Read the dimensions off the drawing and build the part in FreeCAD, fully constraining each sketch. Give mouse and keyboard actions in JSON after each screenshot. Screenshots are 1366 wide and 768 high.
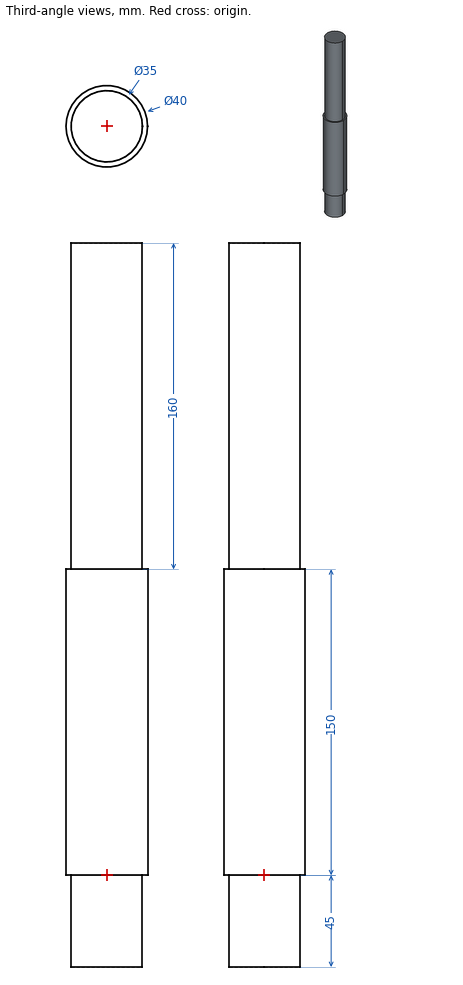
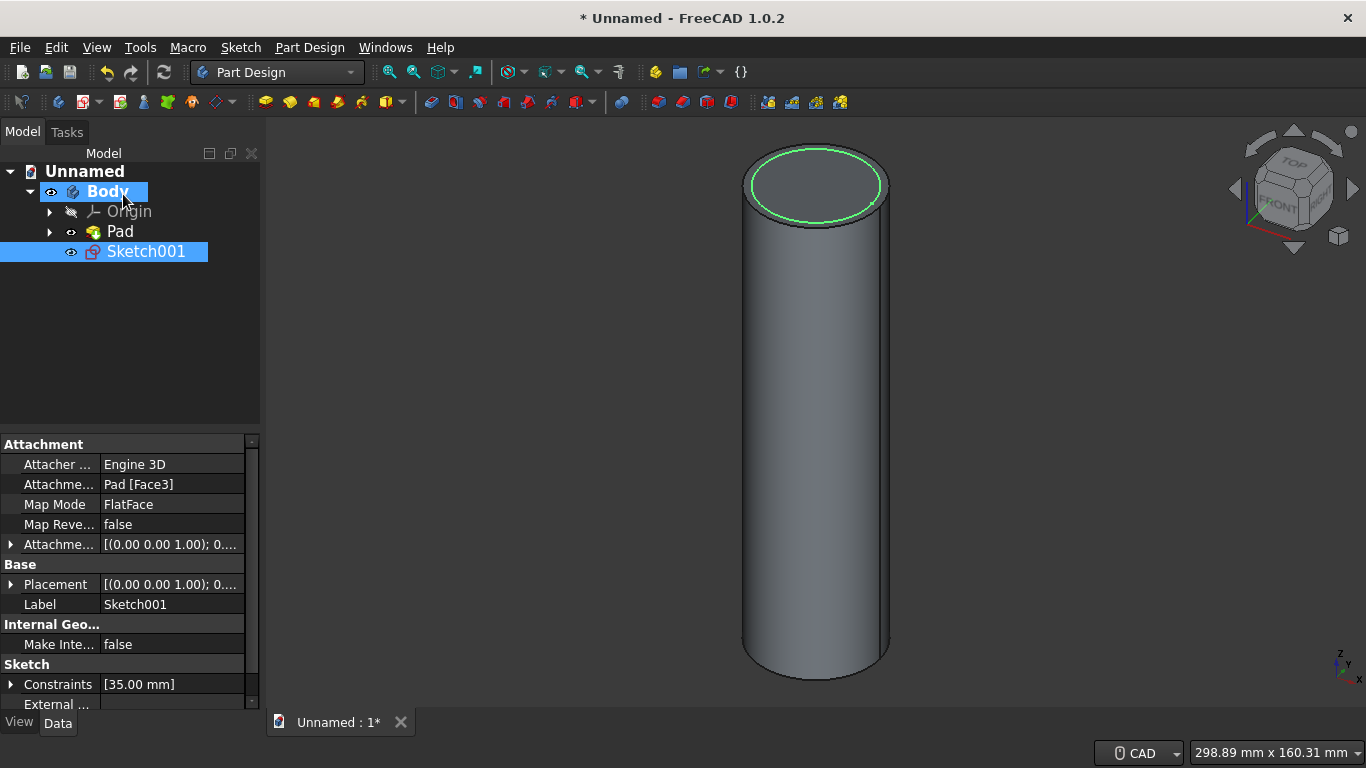
{"action": "left_click", "coordinate": [266, 102]}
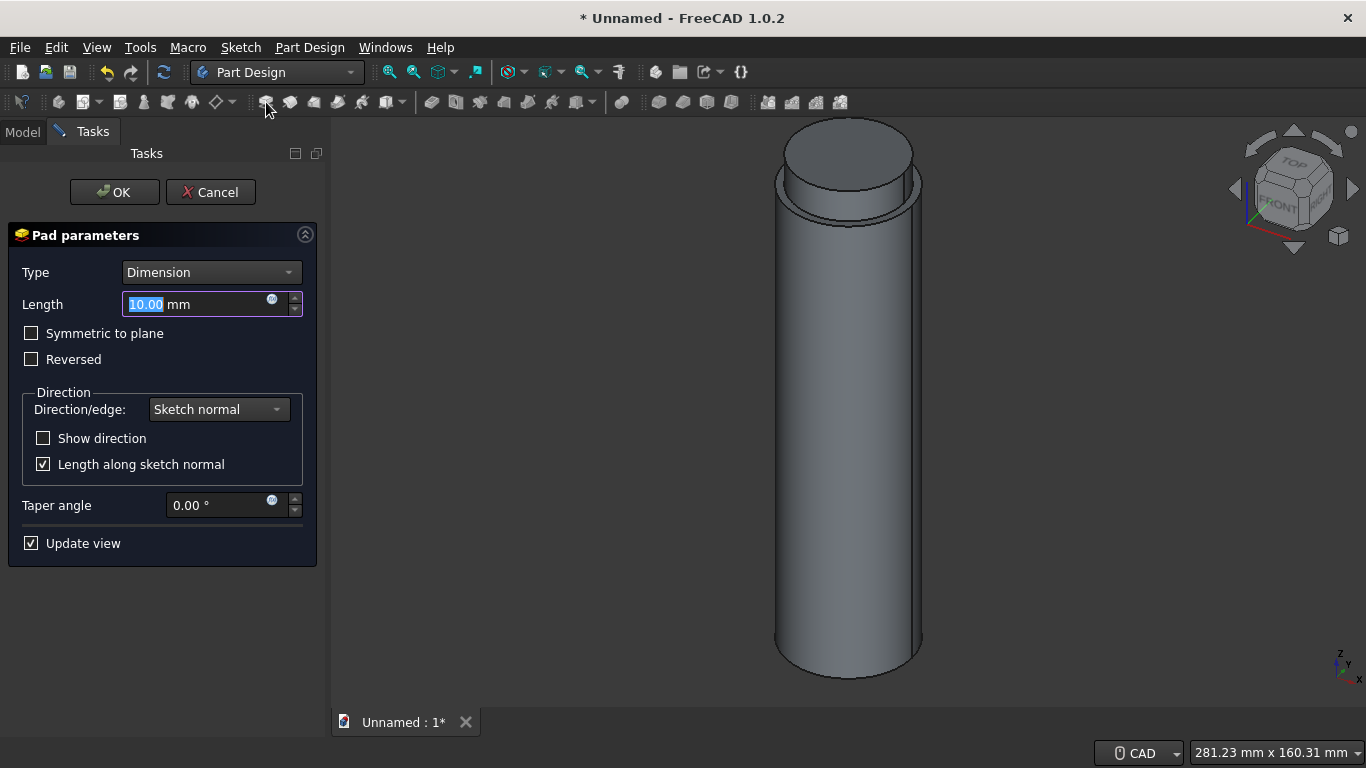
{"action": "type", "text": "160"}
{"action": "key", "text": "Tab"}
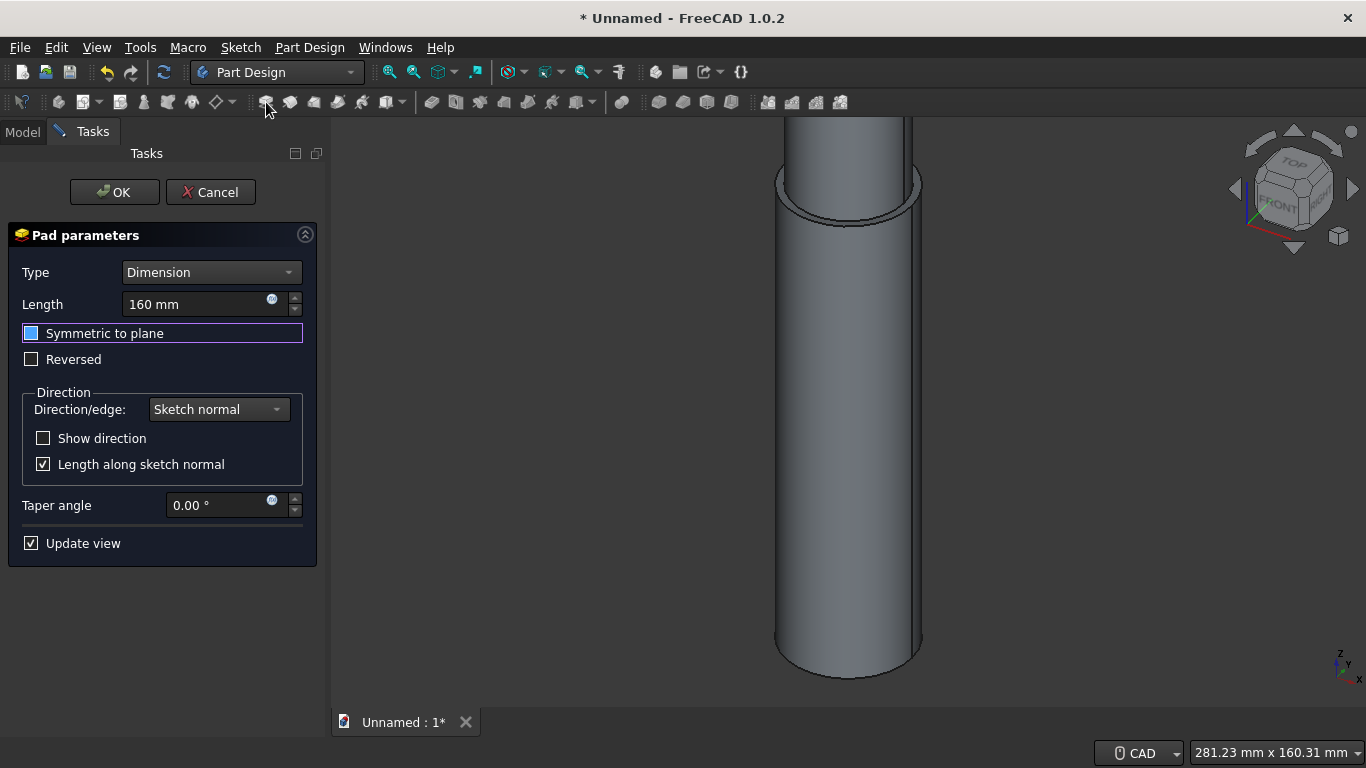
{"action": "left_click", "coordinate": [115, 192]}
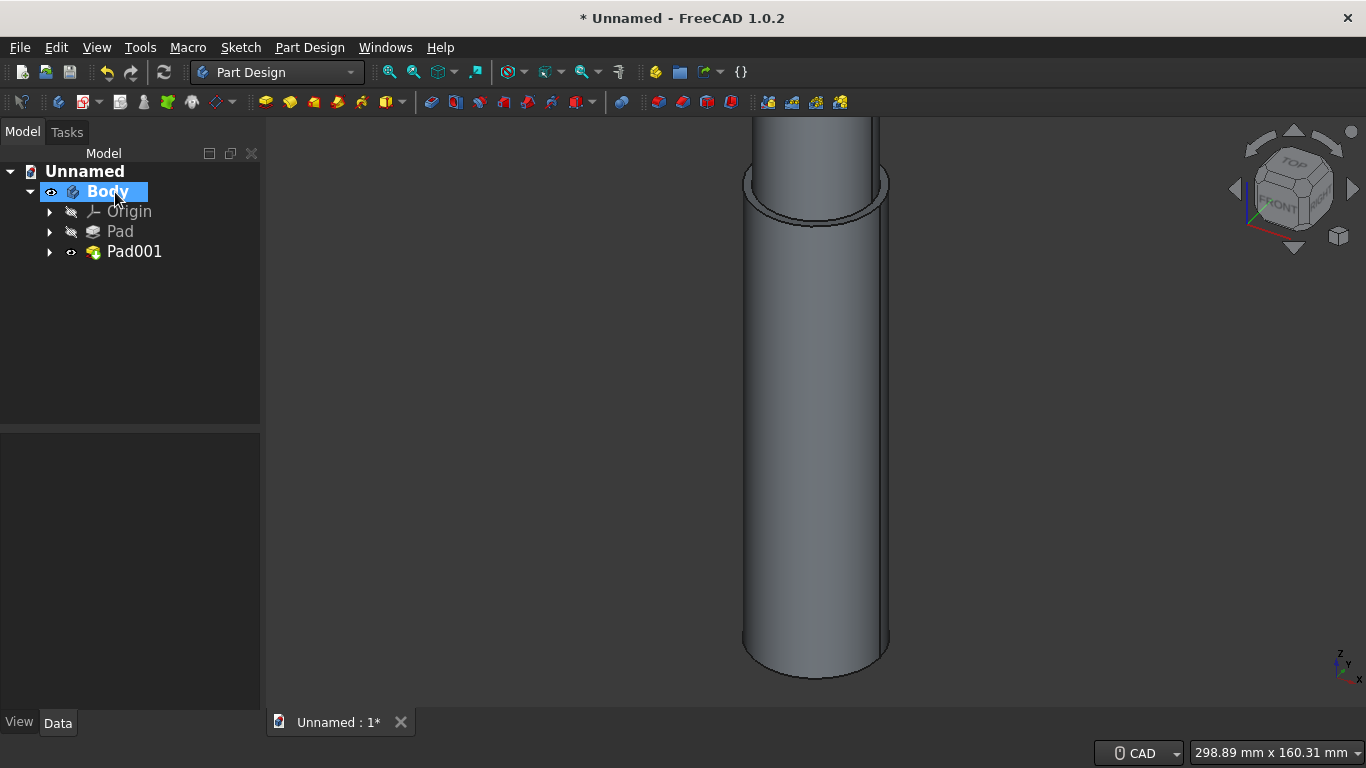
{"action": "left_click", "coordinate": [390, 72]}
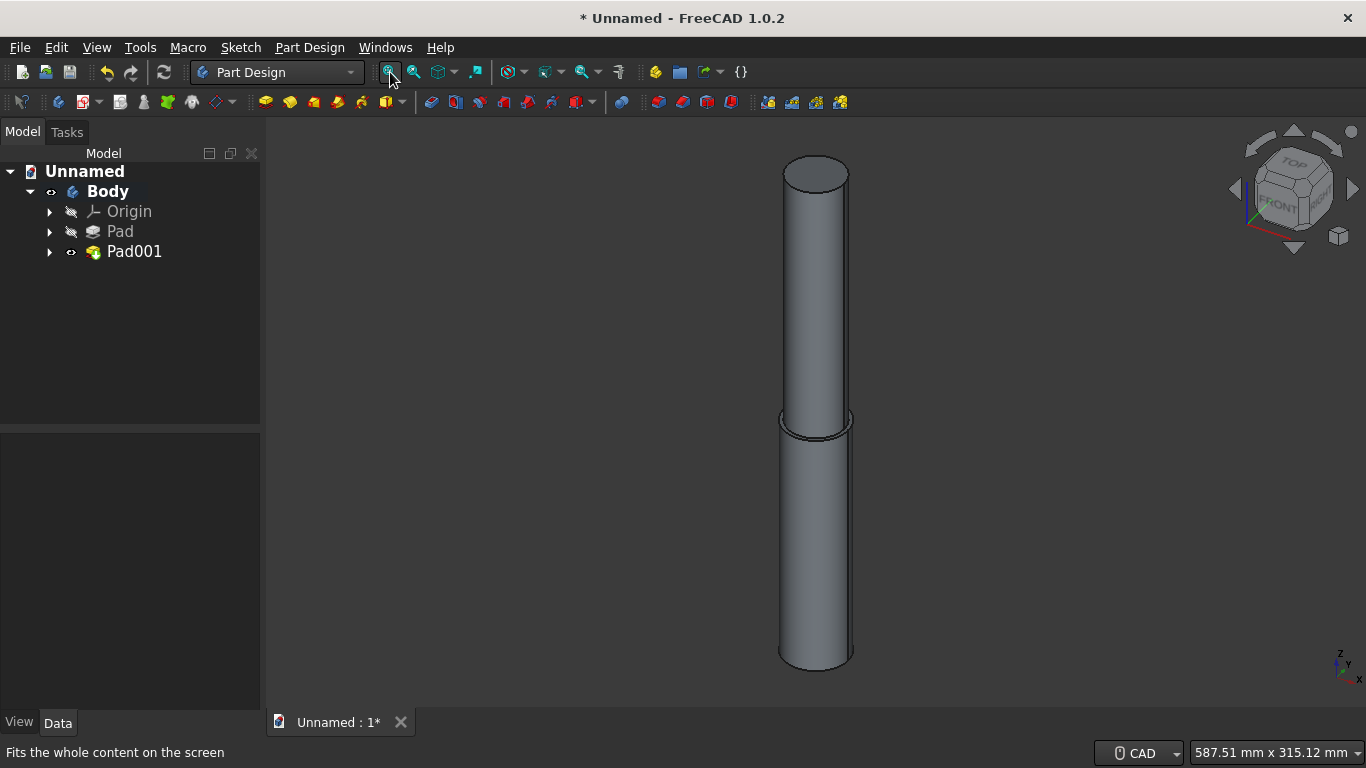
{"action": "left_click", "coordinate": [50, 212]}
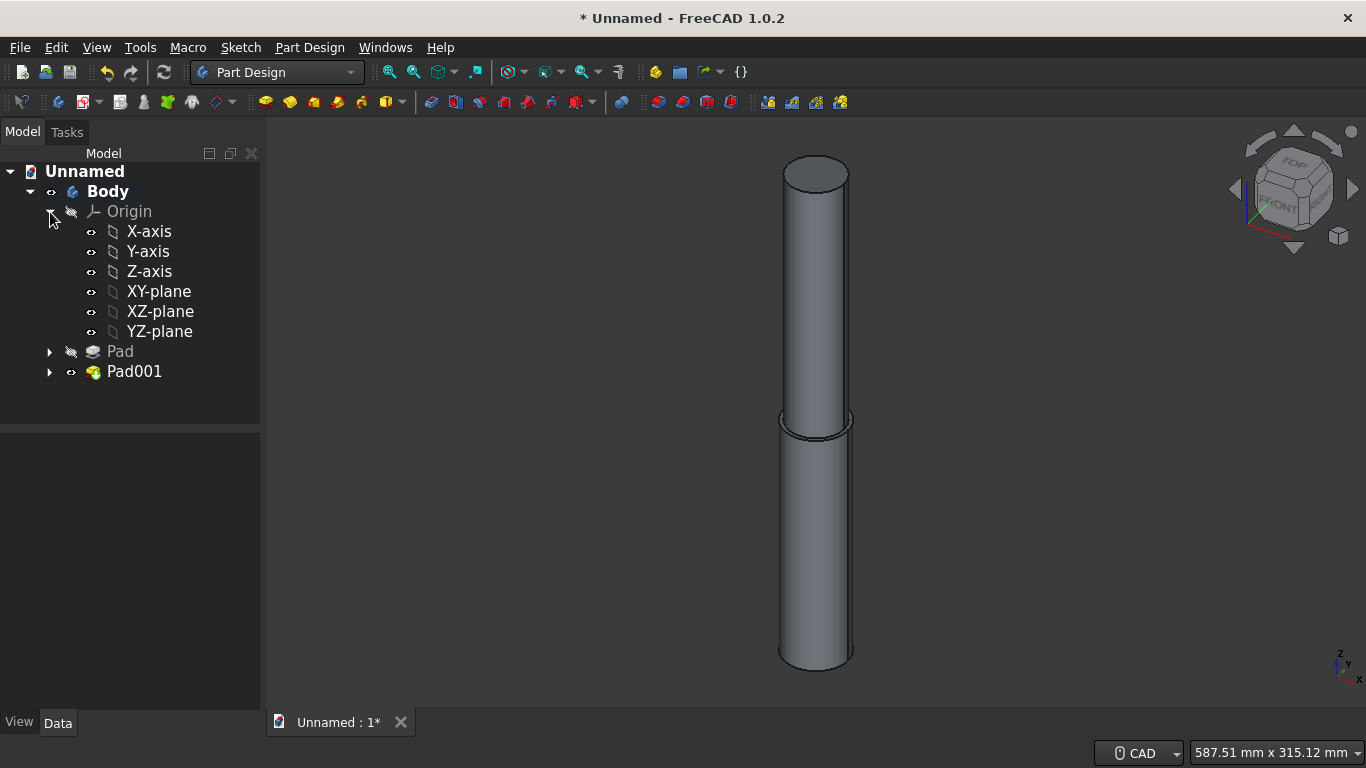
{"action": "left_click", "coordinate": [136, 292]}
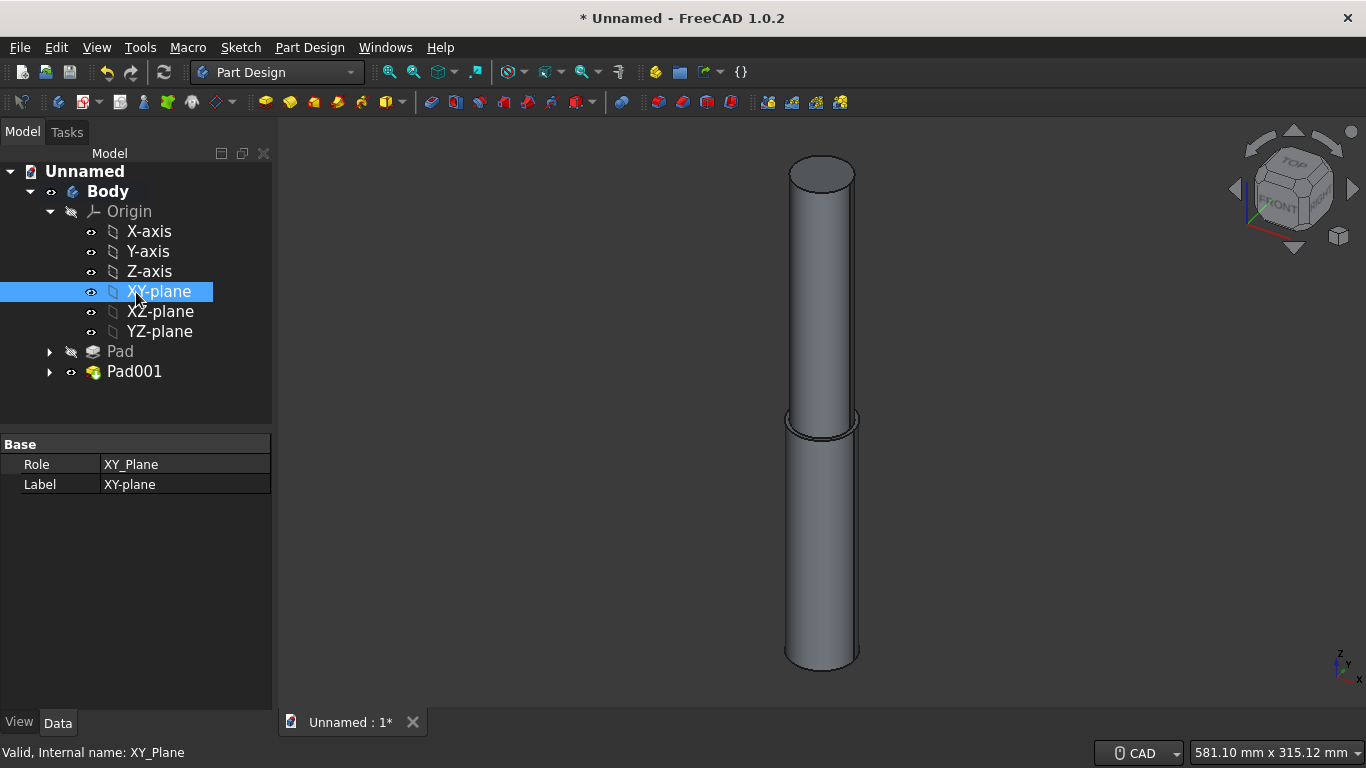
{"action": "left_click", "coordinate": [216, 102]}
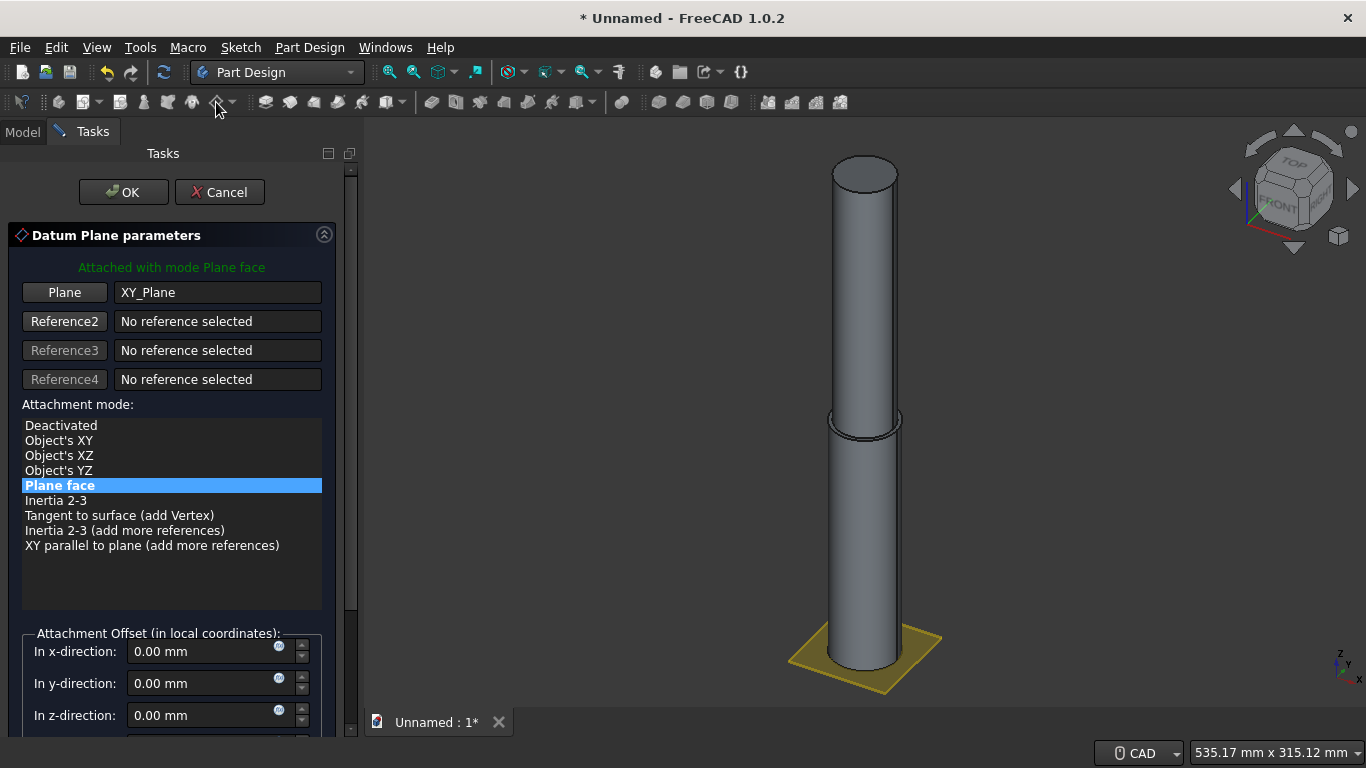
{"action": "triple_click", "coordinate": [210, 715]}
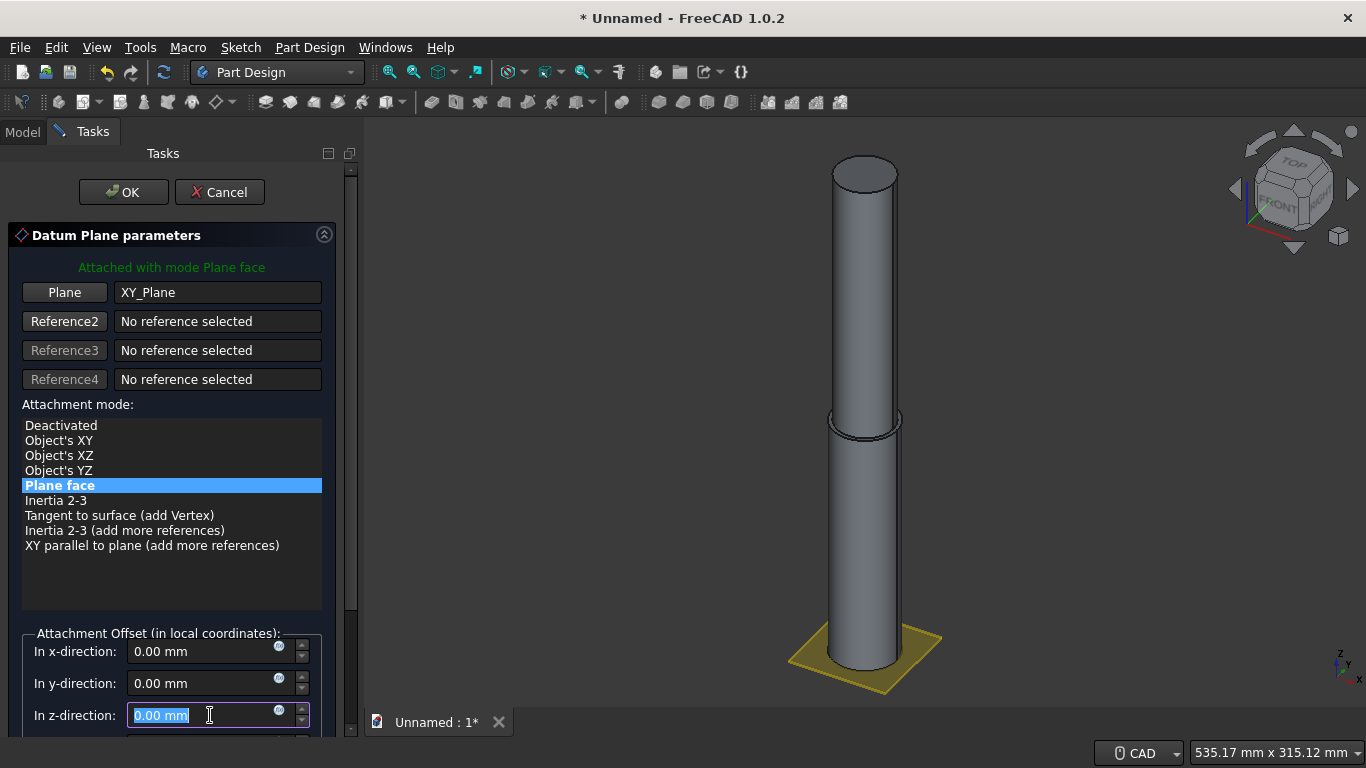
{"action": "type", "text": "-45"}
{"action": "key", "text": "Tab"}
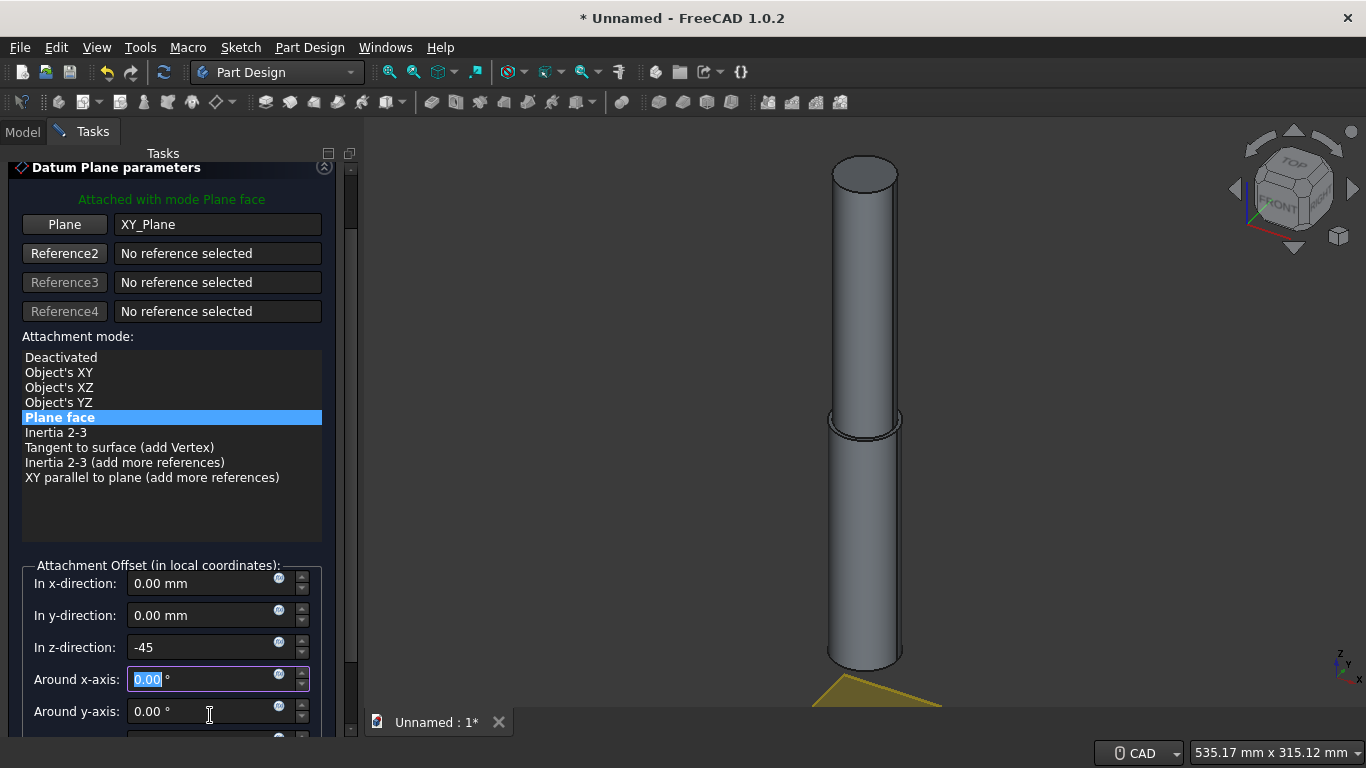
{"action": "scroll", "coordinate": [351, 450], "scroll_direction": "up", "scroll_amount": 2}